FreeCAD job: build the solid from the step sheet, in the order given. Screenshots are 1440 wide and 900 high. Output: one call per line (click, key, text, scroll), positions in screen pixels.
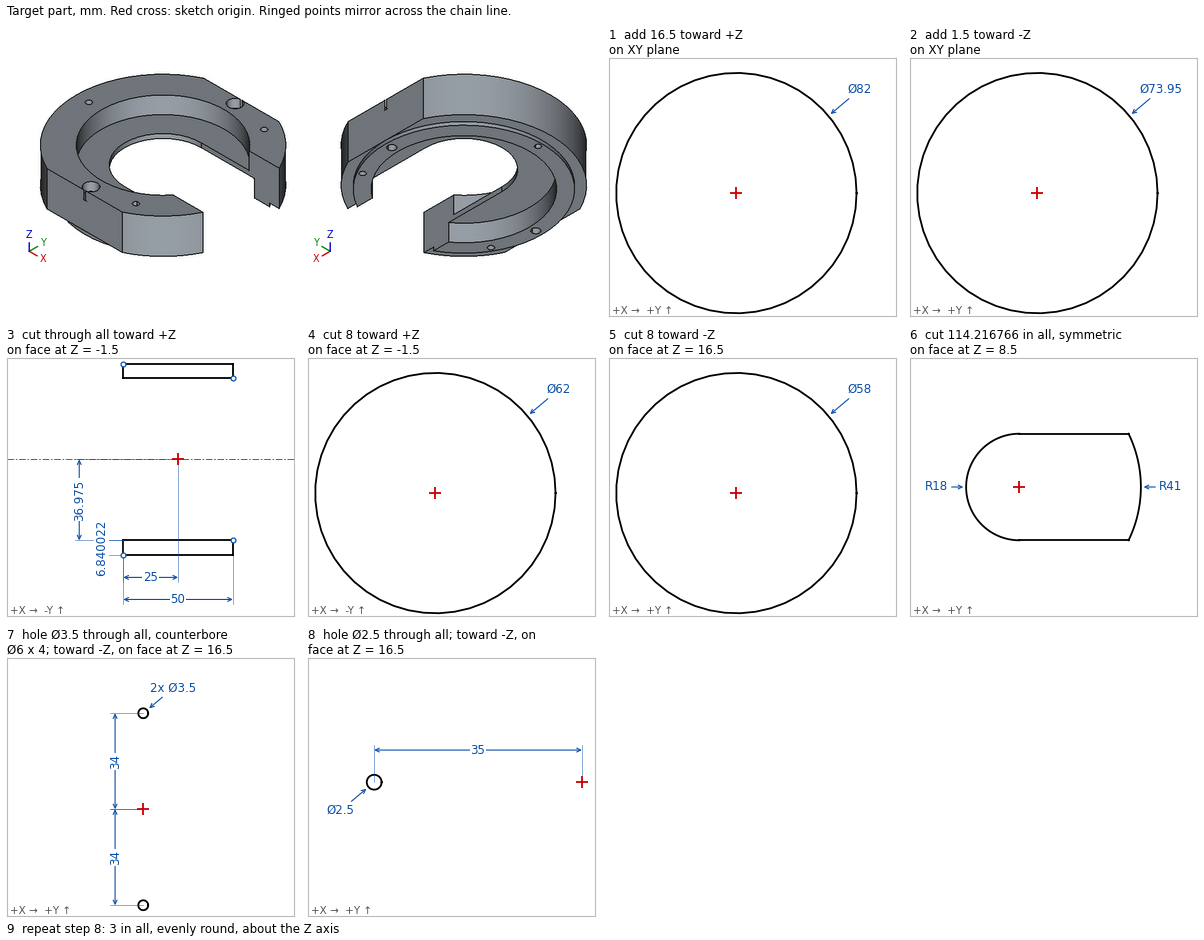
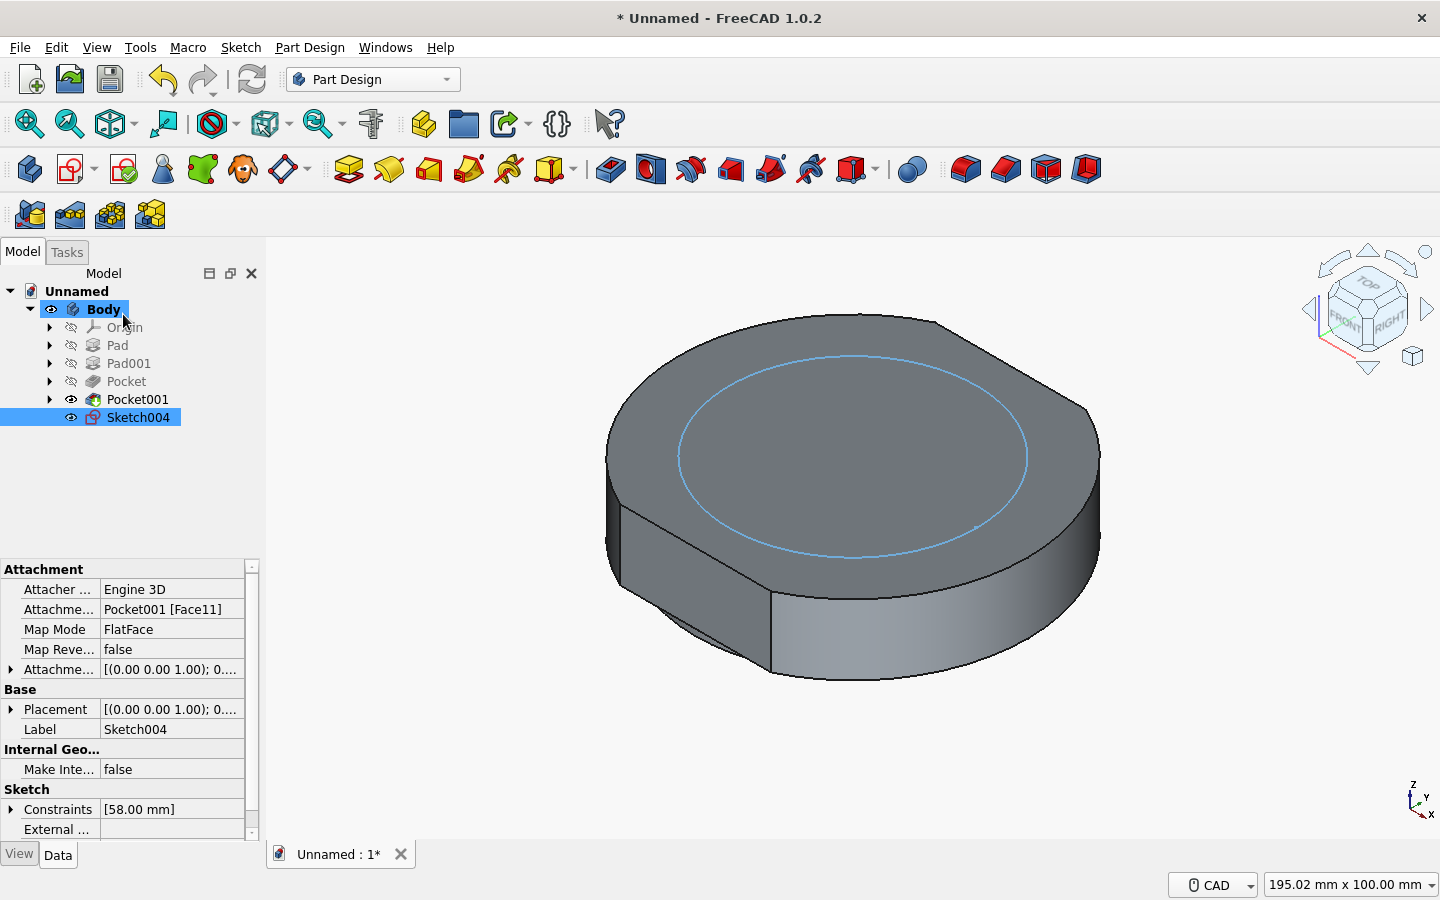
click(612, 170)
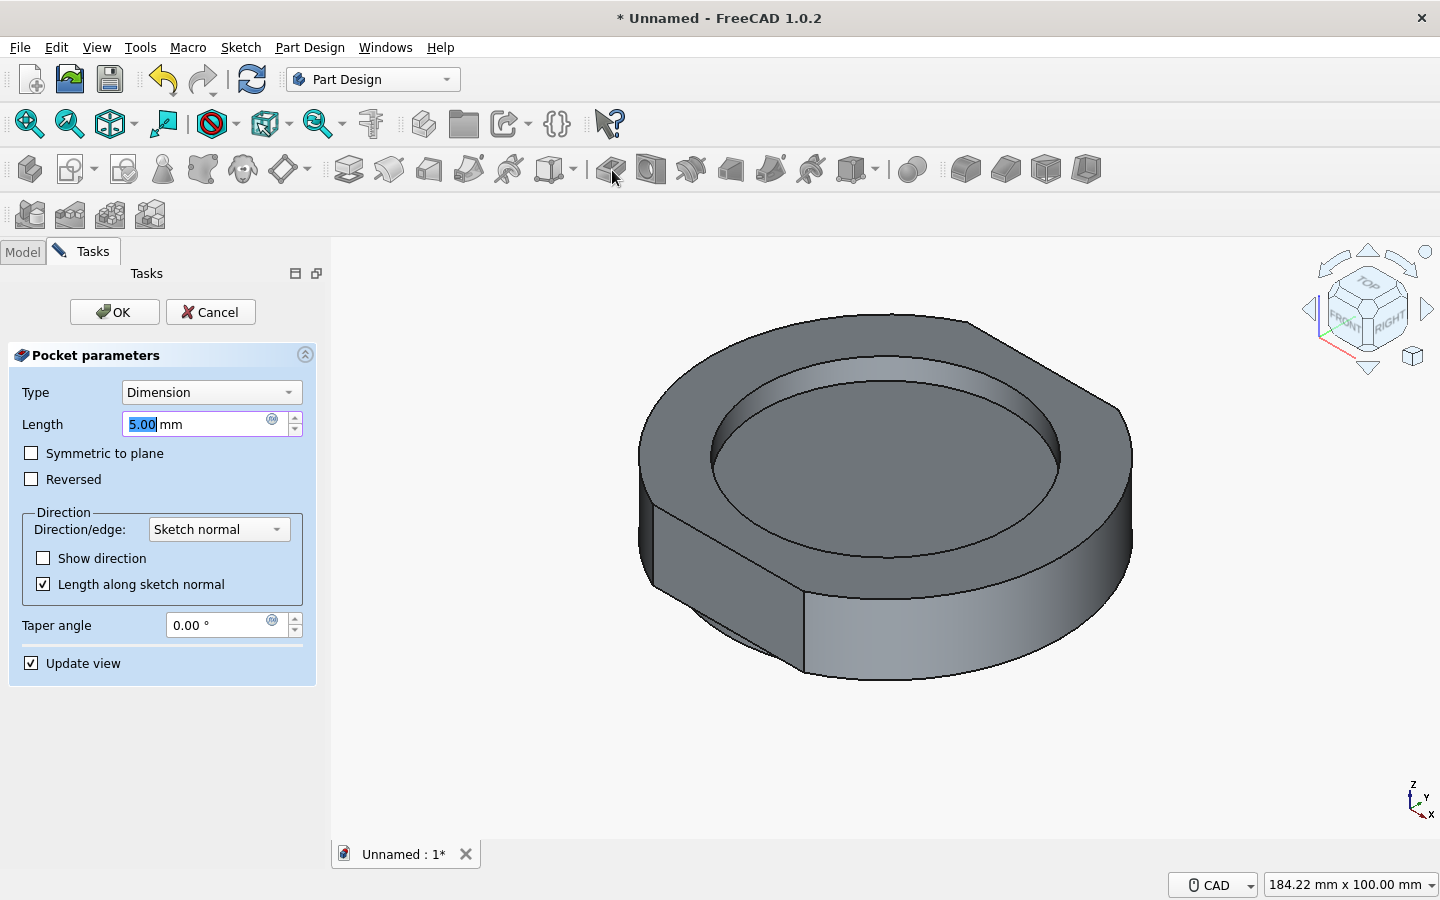
text(8)
key(Tab)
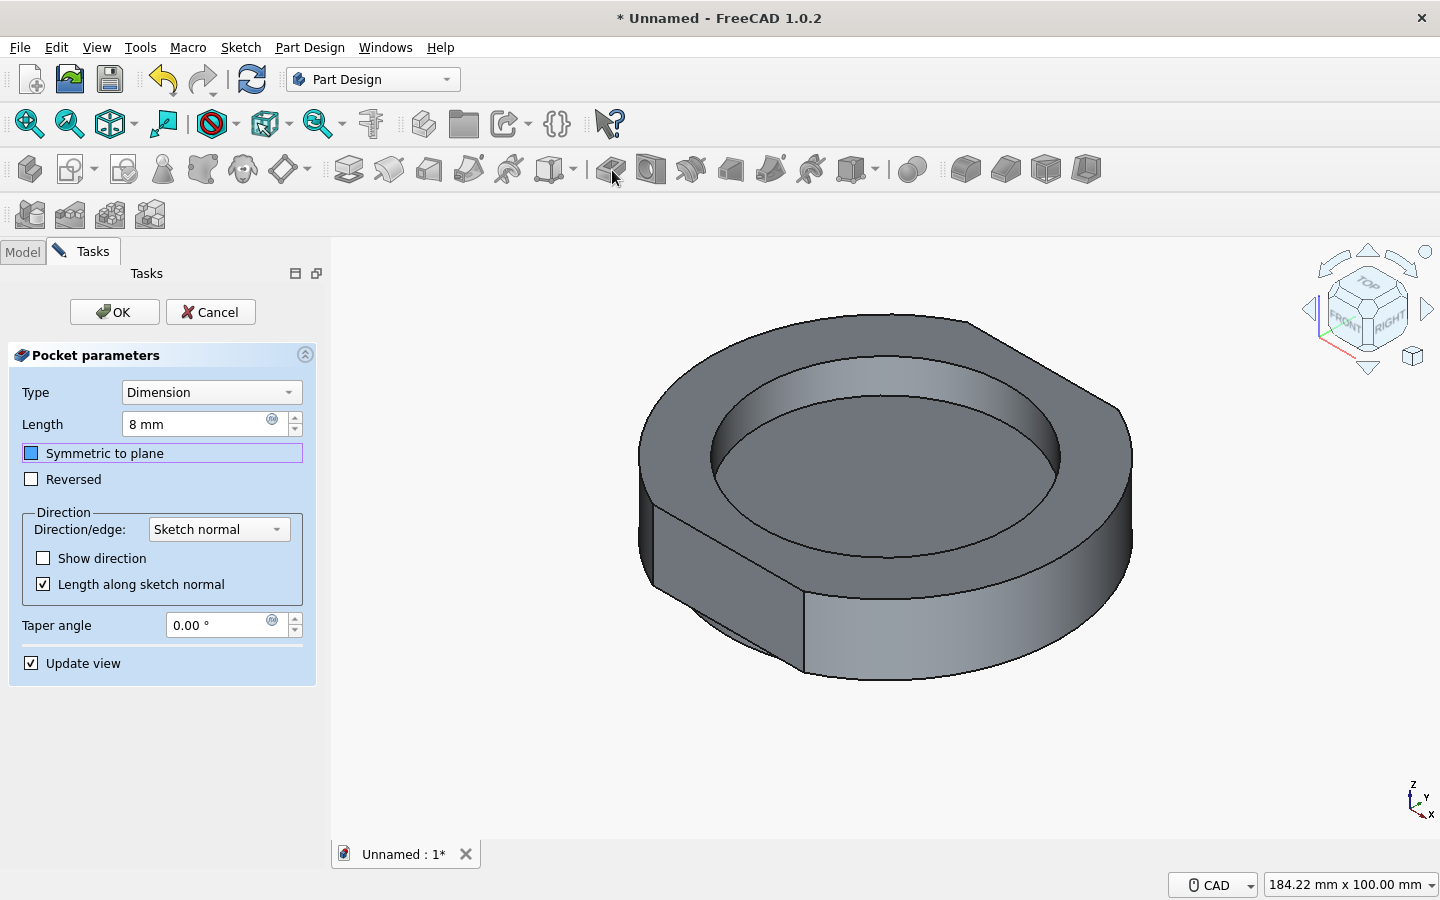
click(115, 312)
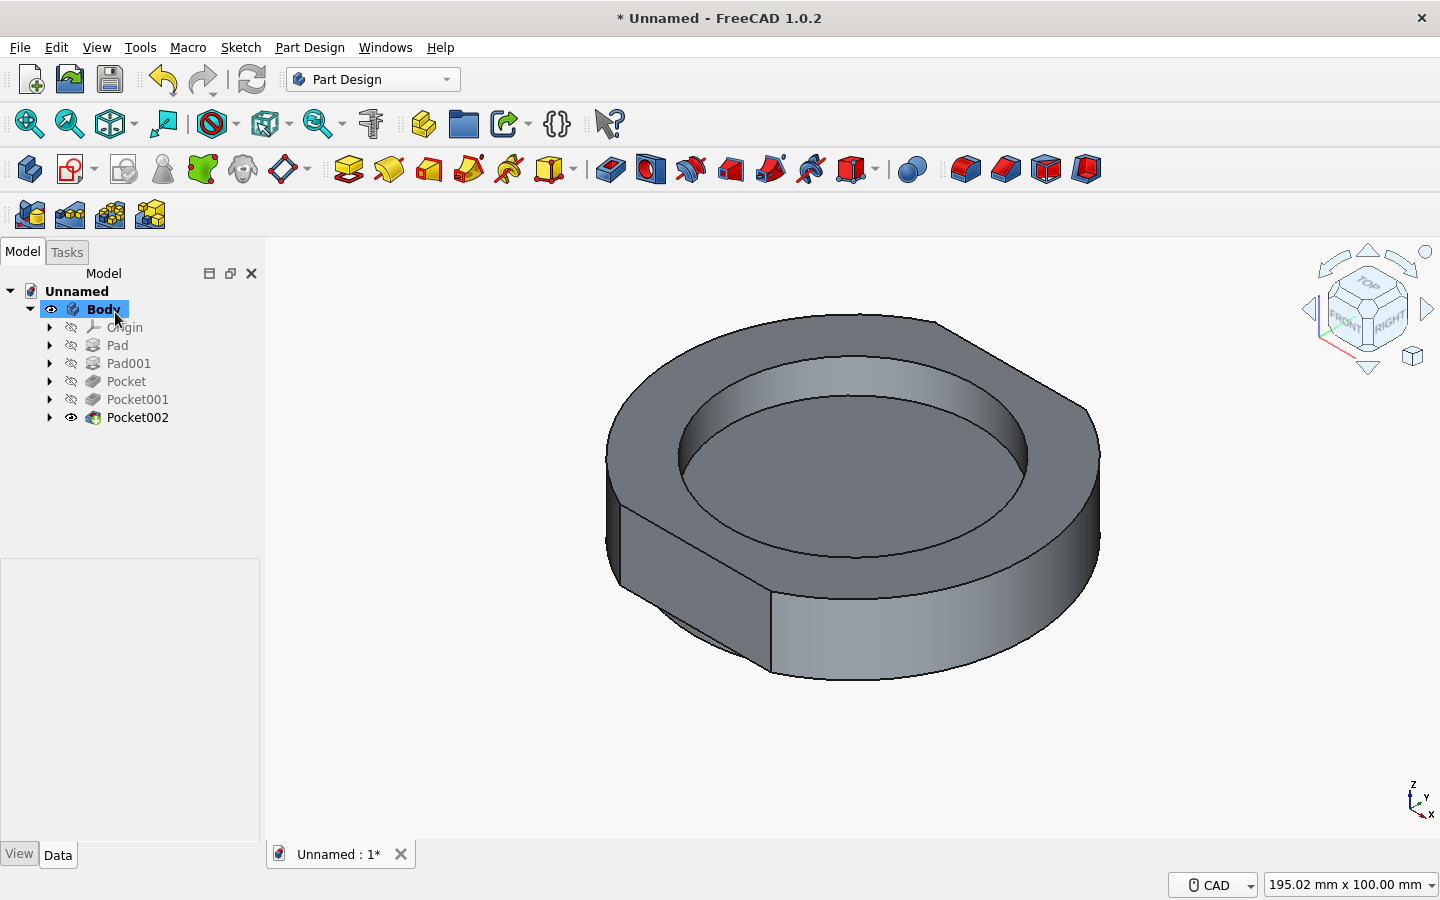
click(853, 495)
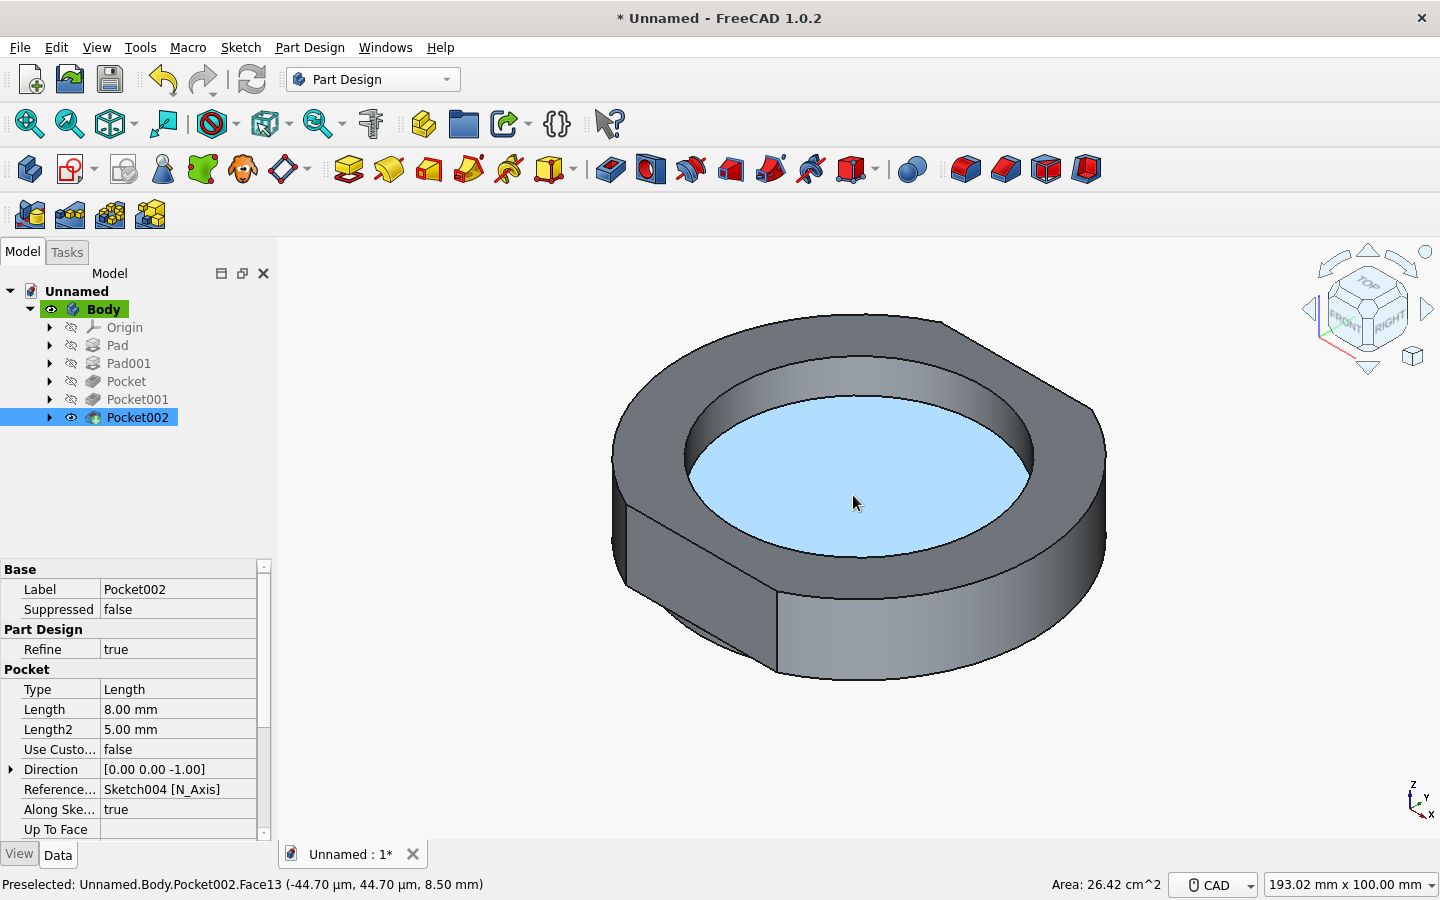
click(70, 170)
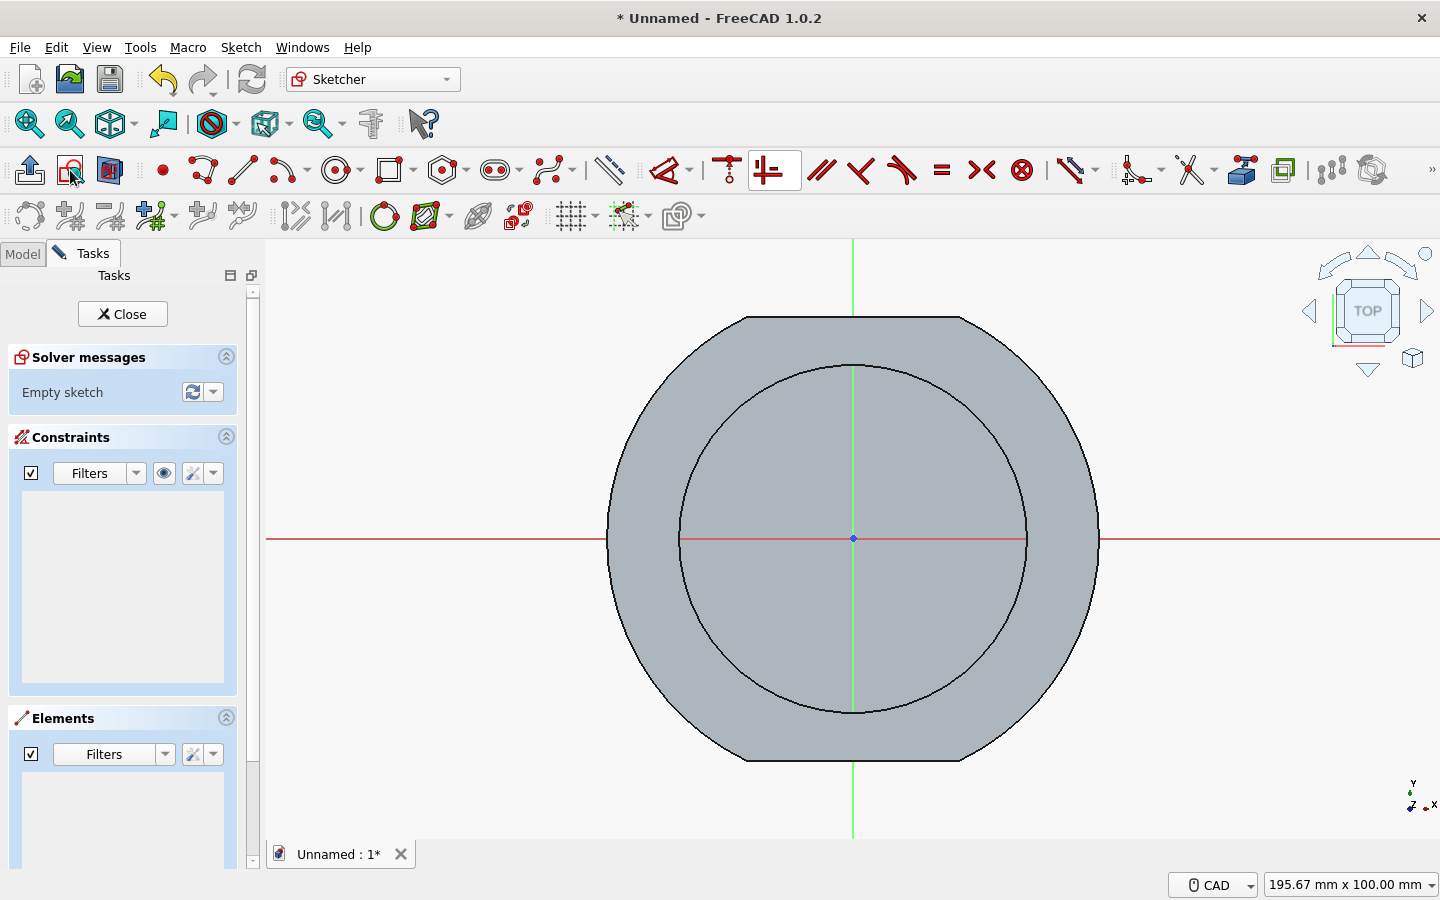
key(q)
key(s)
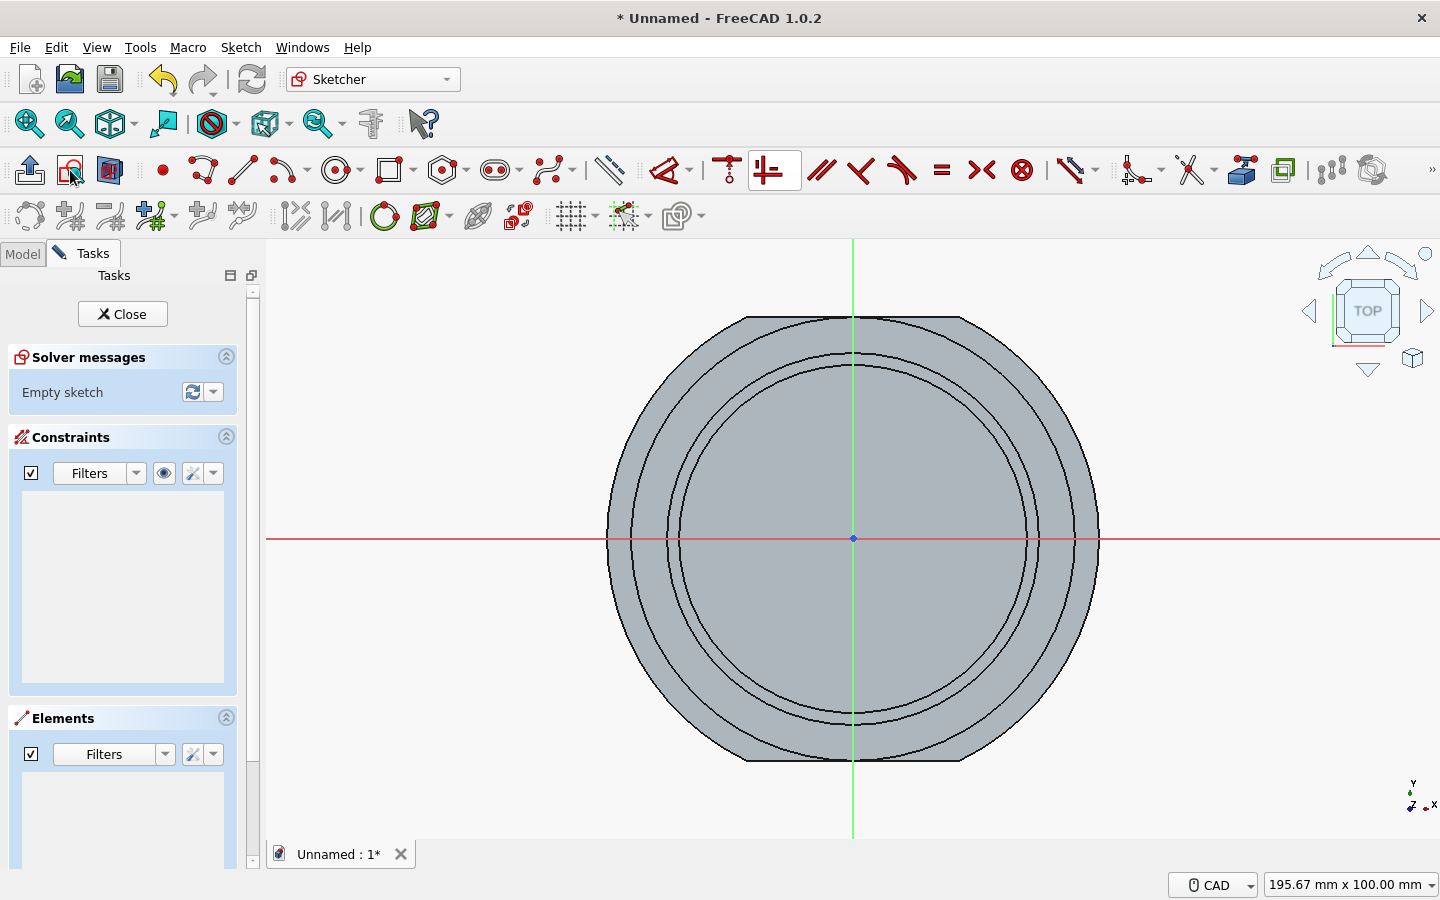
scroll(1089, 539, up, 3)